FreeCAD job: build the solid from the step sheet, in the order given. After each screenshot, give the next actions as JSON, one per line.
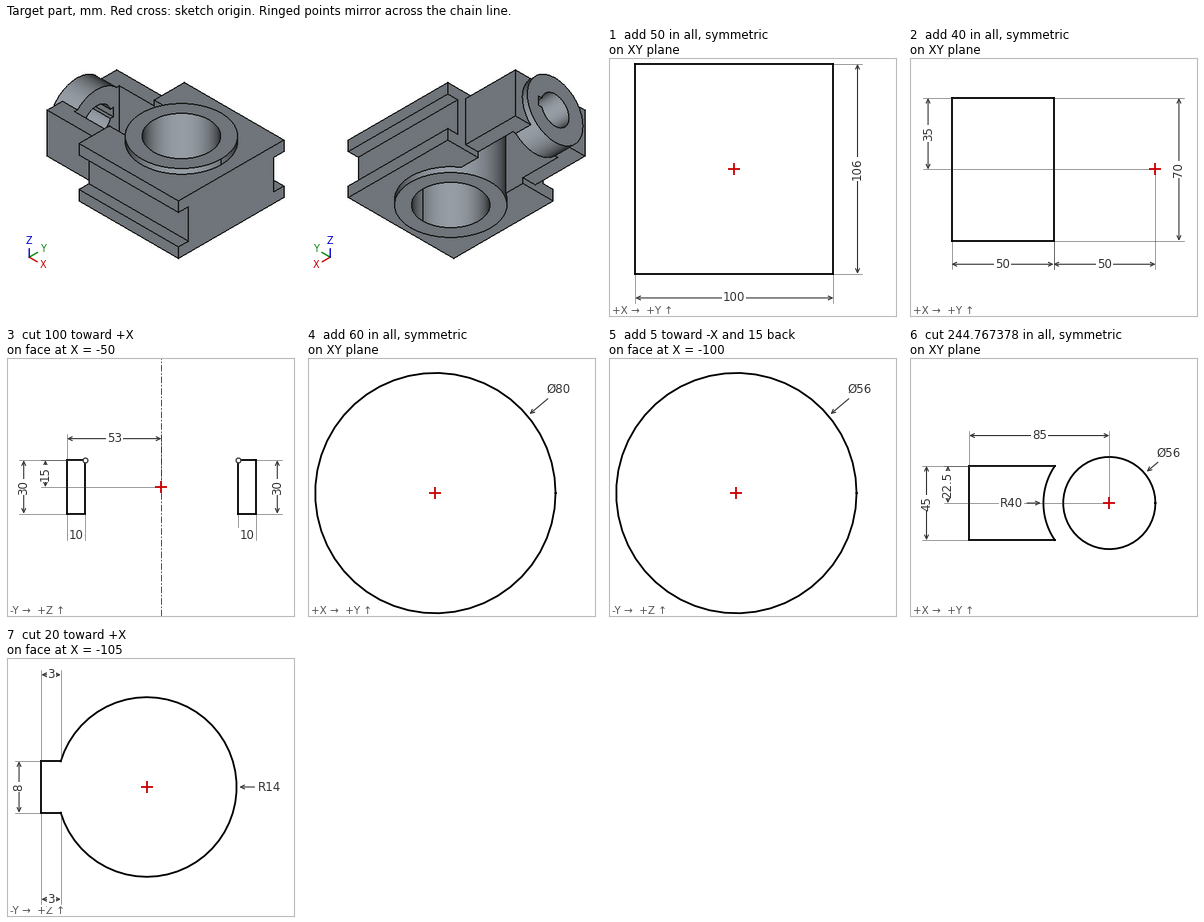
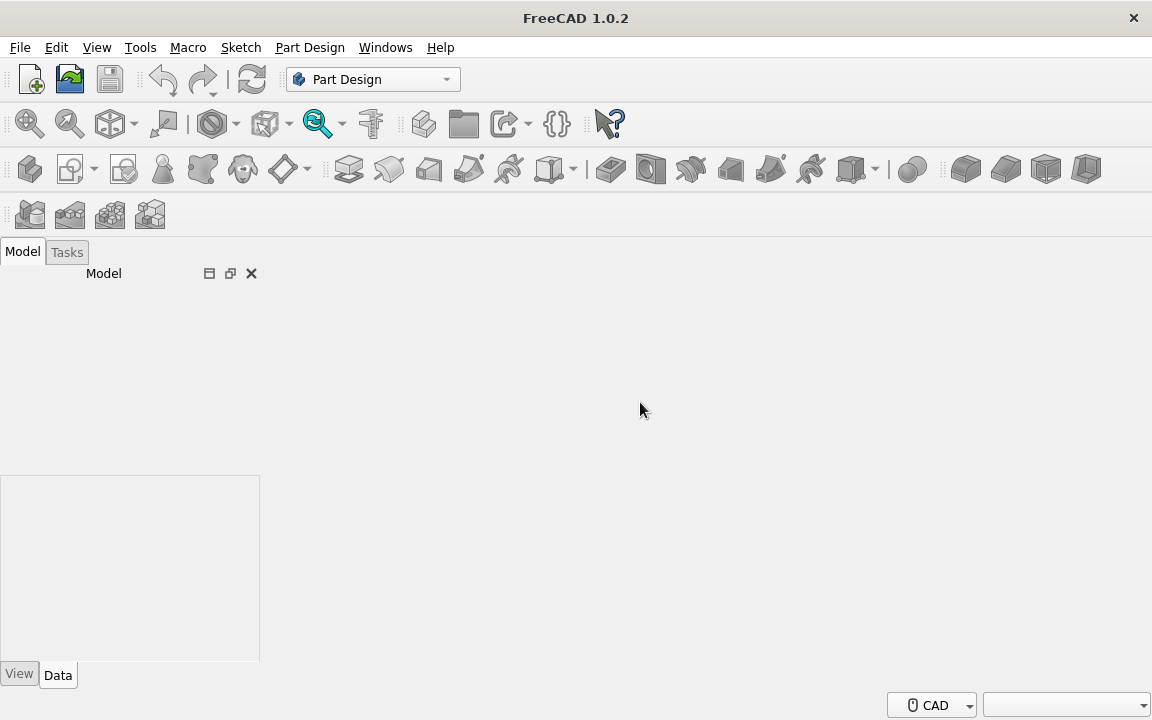
{"action": "left_click", "coordinate": [30, 80]}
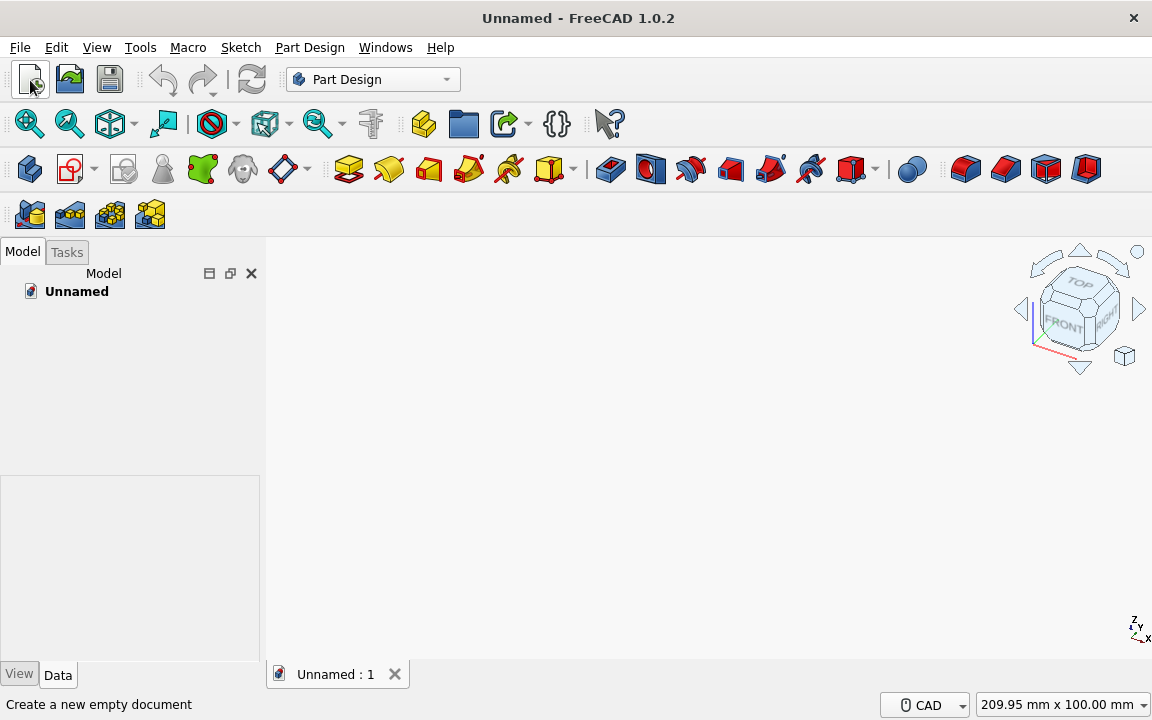
{"action": "left_click", "coordinate": [70, 170]}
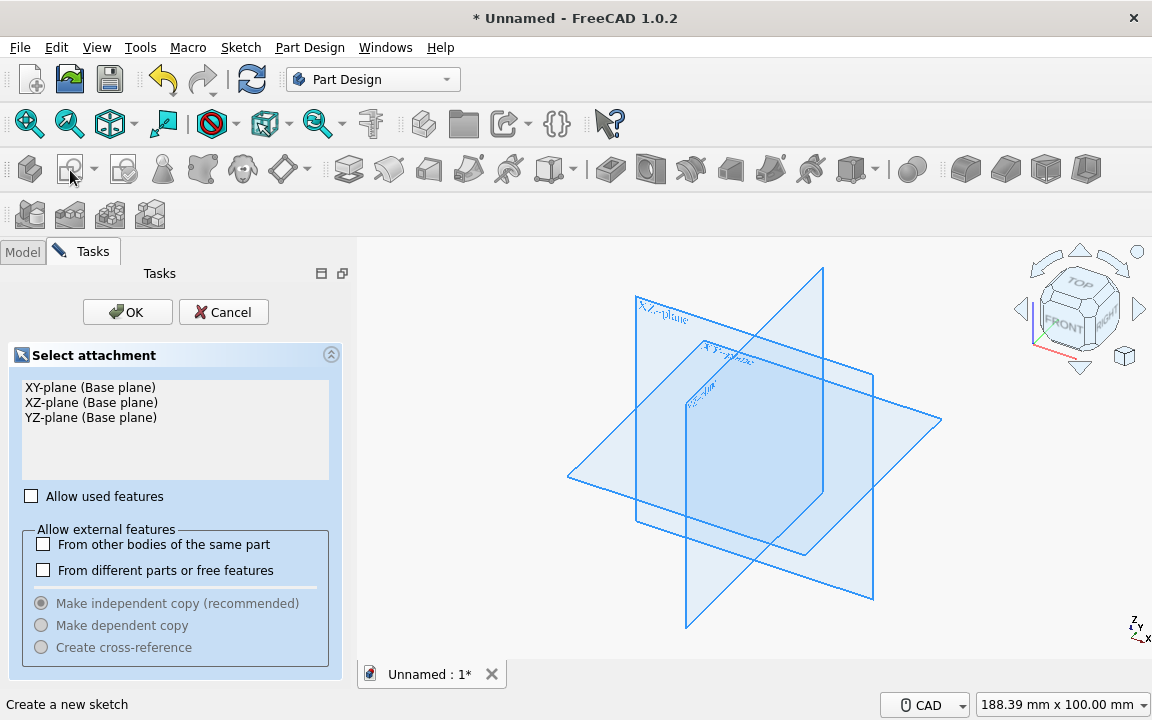
{"action": "left_click", "coordinate": [82, 388]}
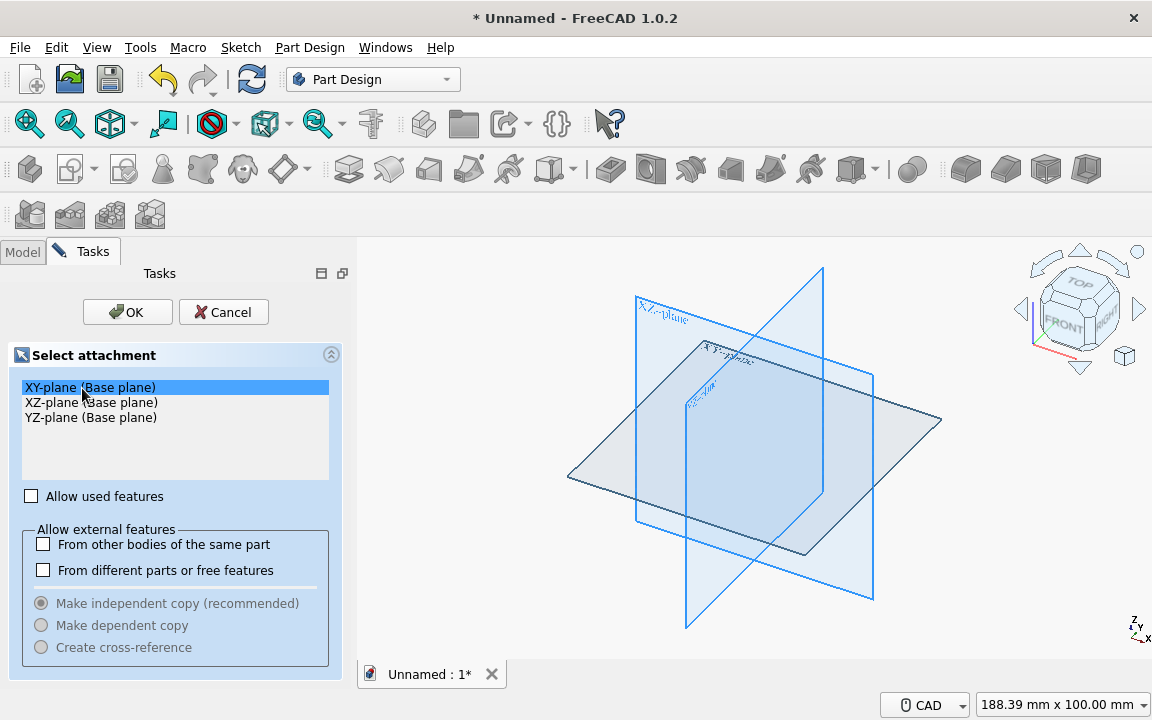
{"action": "left_click", "coordinate": [128, 312]}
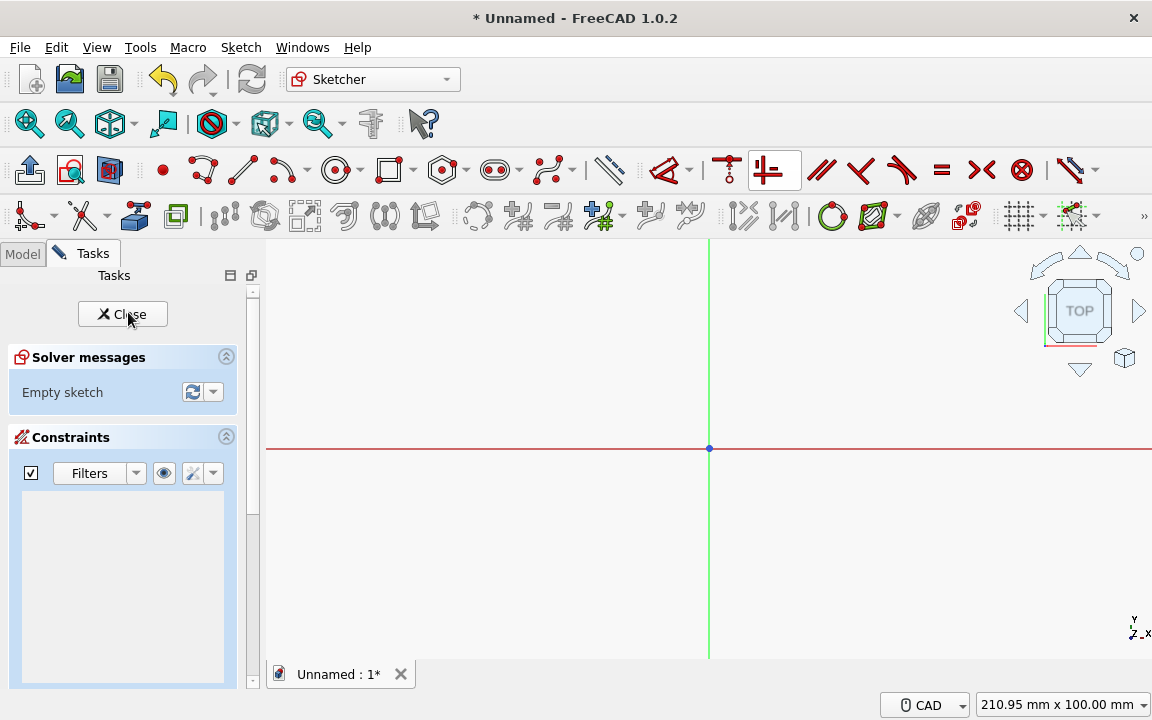
{"action": "scroll", "coordinate": [557, 449], "scroll_direction": "down", "scroll_amount": 3}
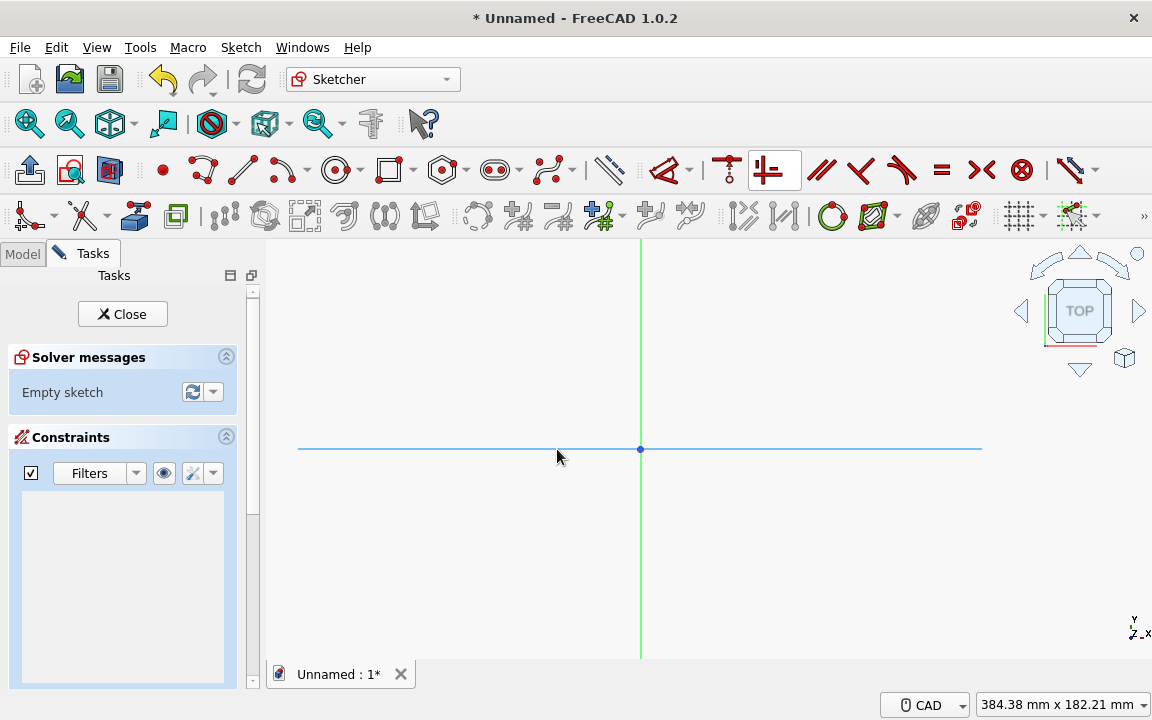
{"action": "key", "text": "g v"}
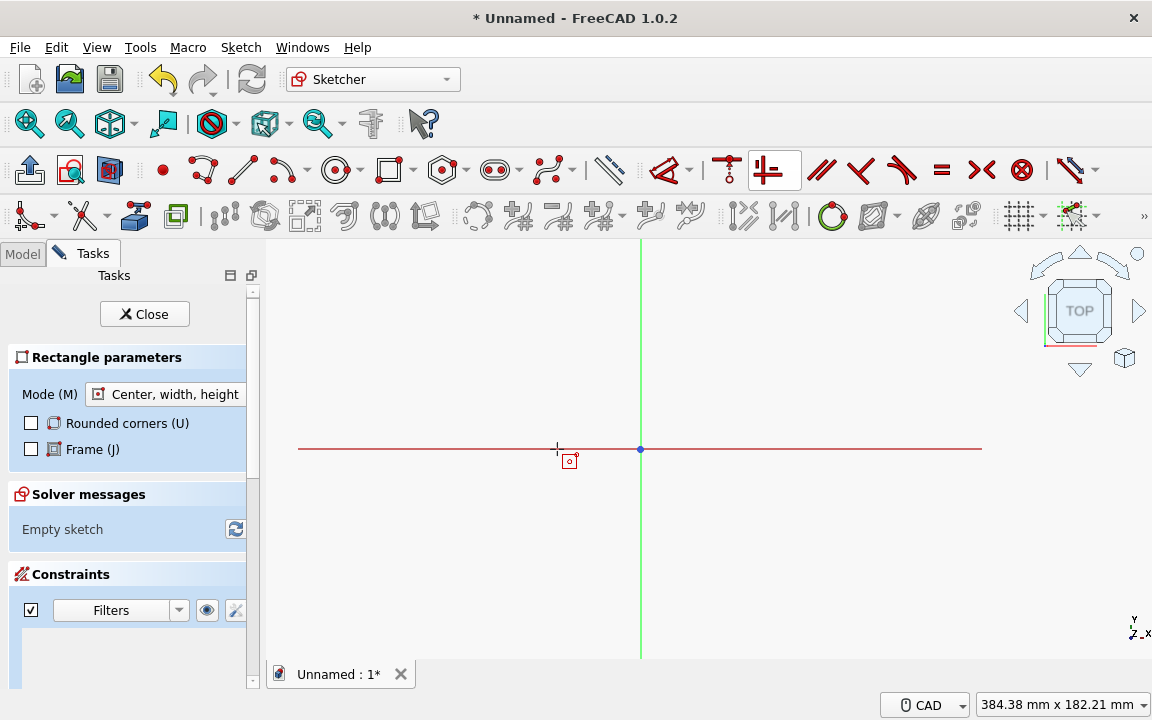
{"action": "left_click", "coordinate": [641, 449]}
{"action": "mouse_move", "coordinate": [756, 327]}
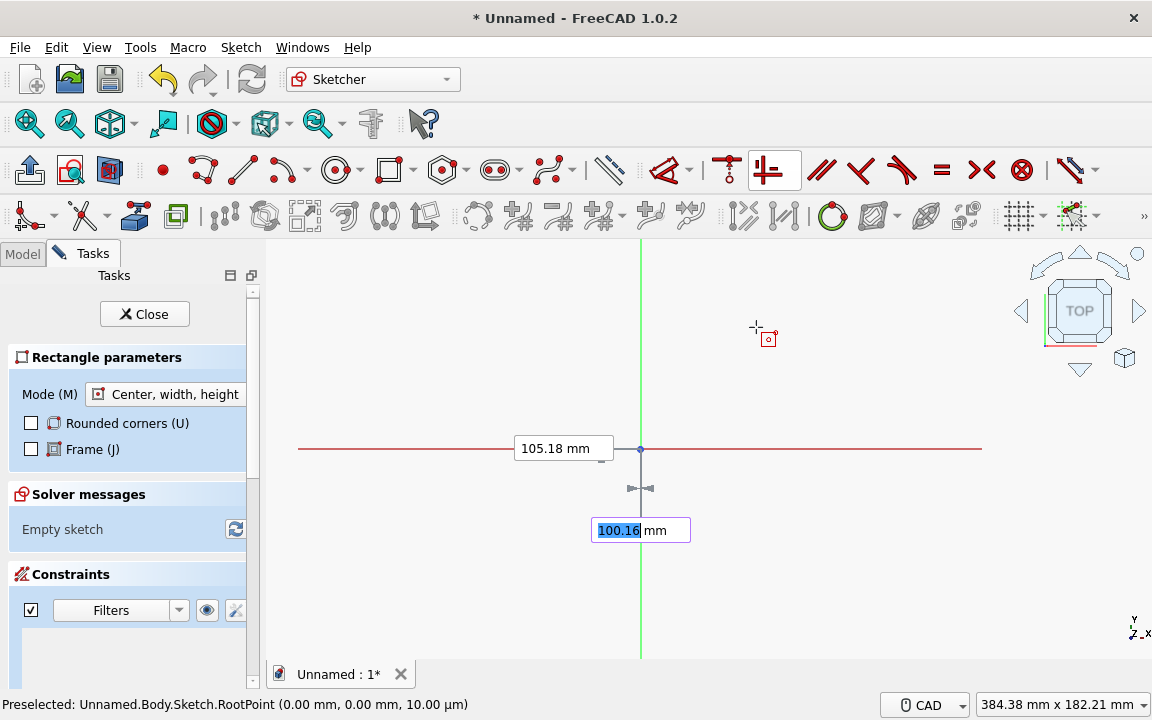
{"action": "type", "text": "100"}
{"action": "key", "text": "Tab"}
{"action": "type", "text": "106"}
{"action": "key", "text": "Return"}
{"action": "key", "text": "Escape"}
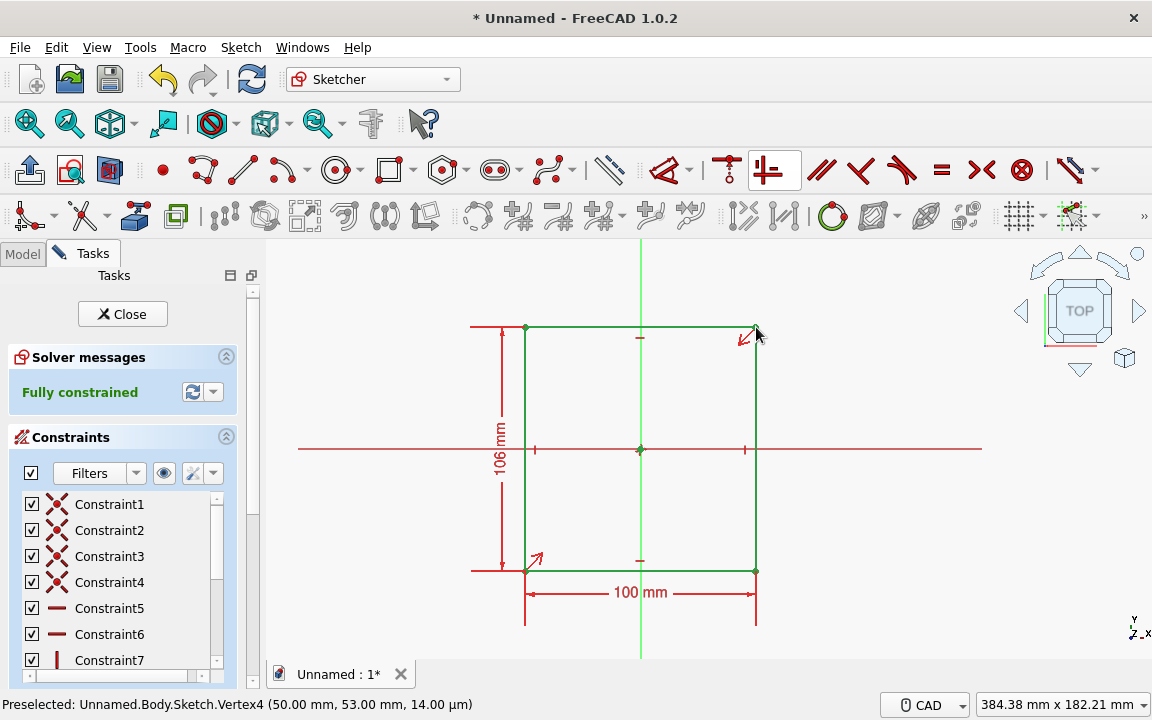
{"action": "left_click", "coordinate": [123, 314]}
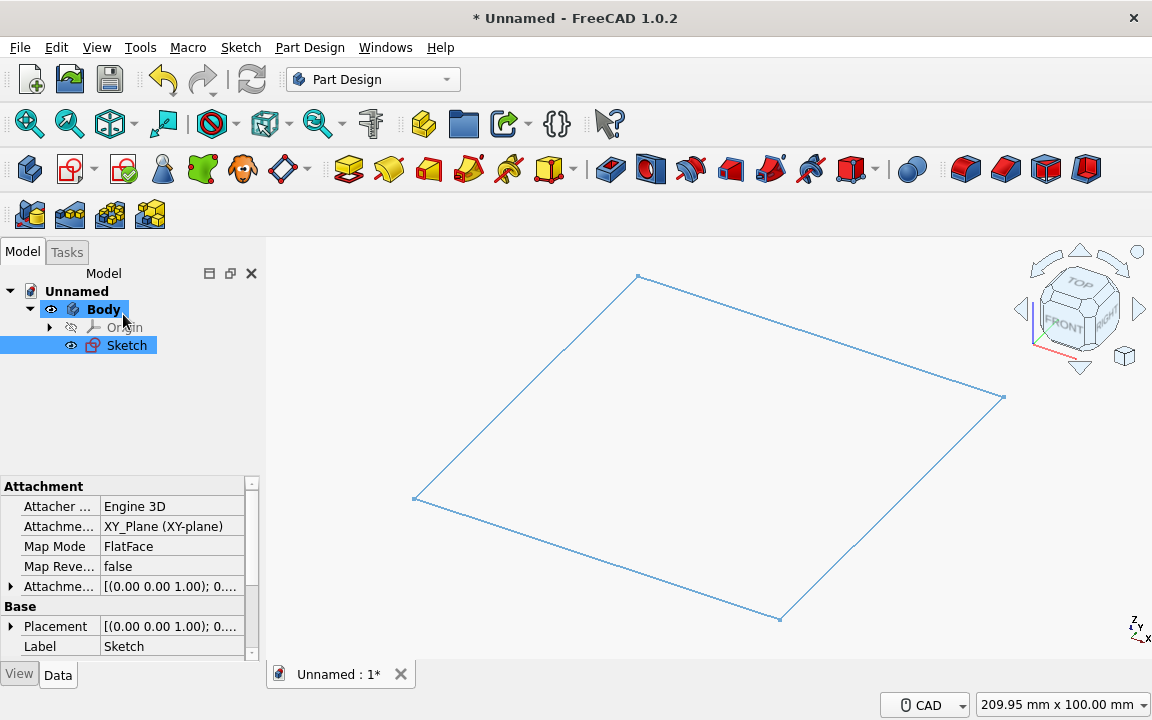
{"action": "left_click", "coordinate": [350, 170]}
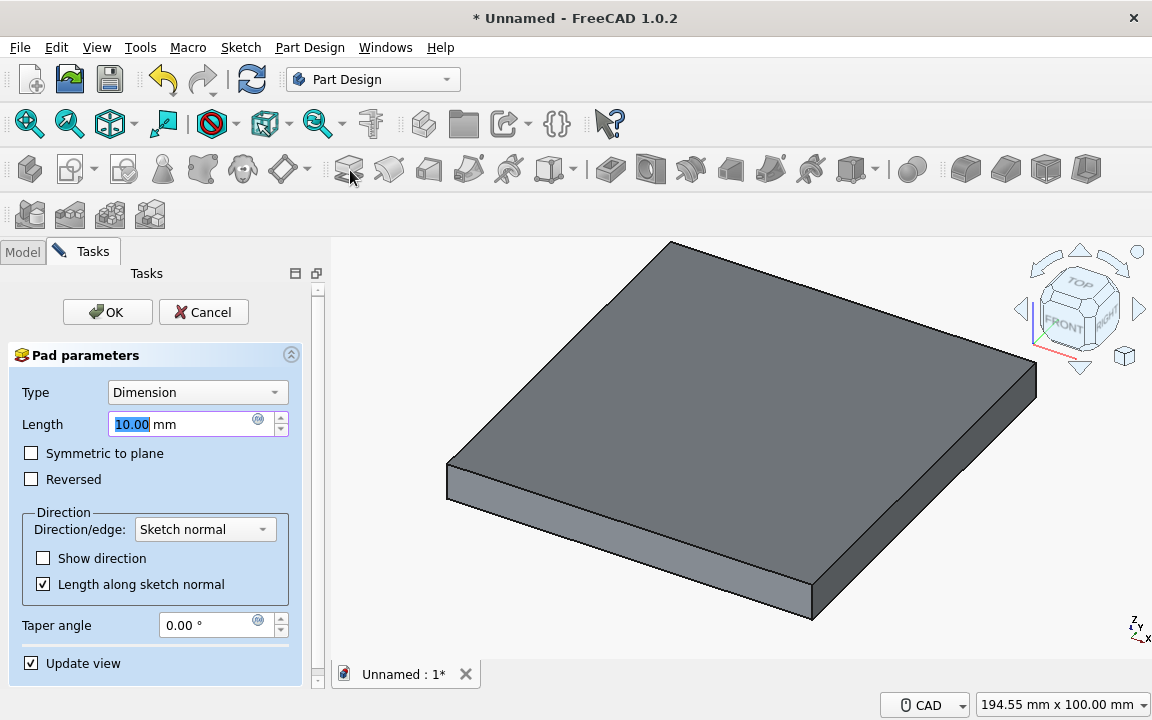
{"action": "type", "text": "50"}
{"action": "key", "text": "Tab"}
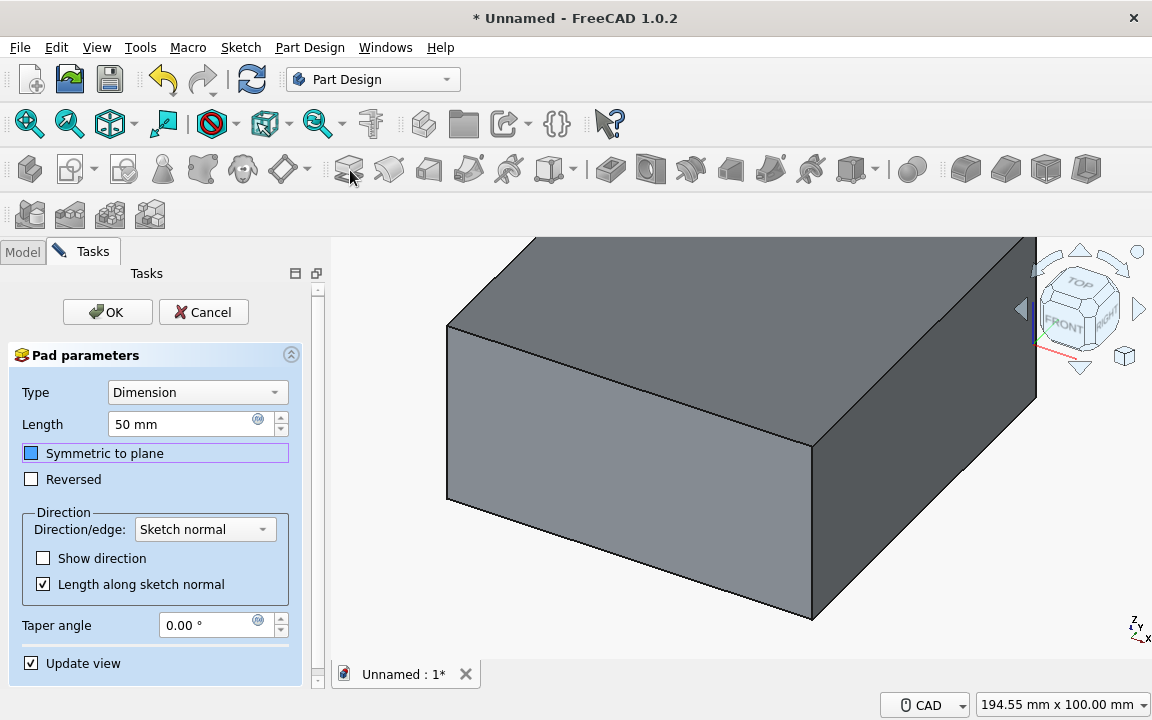
{"action": "left_click", "coordinate": [30, 453]}